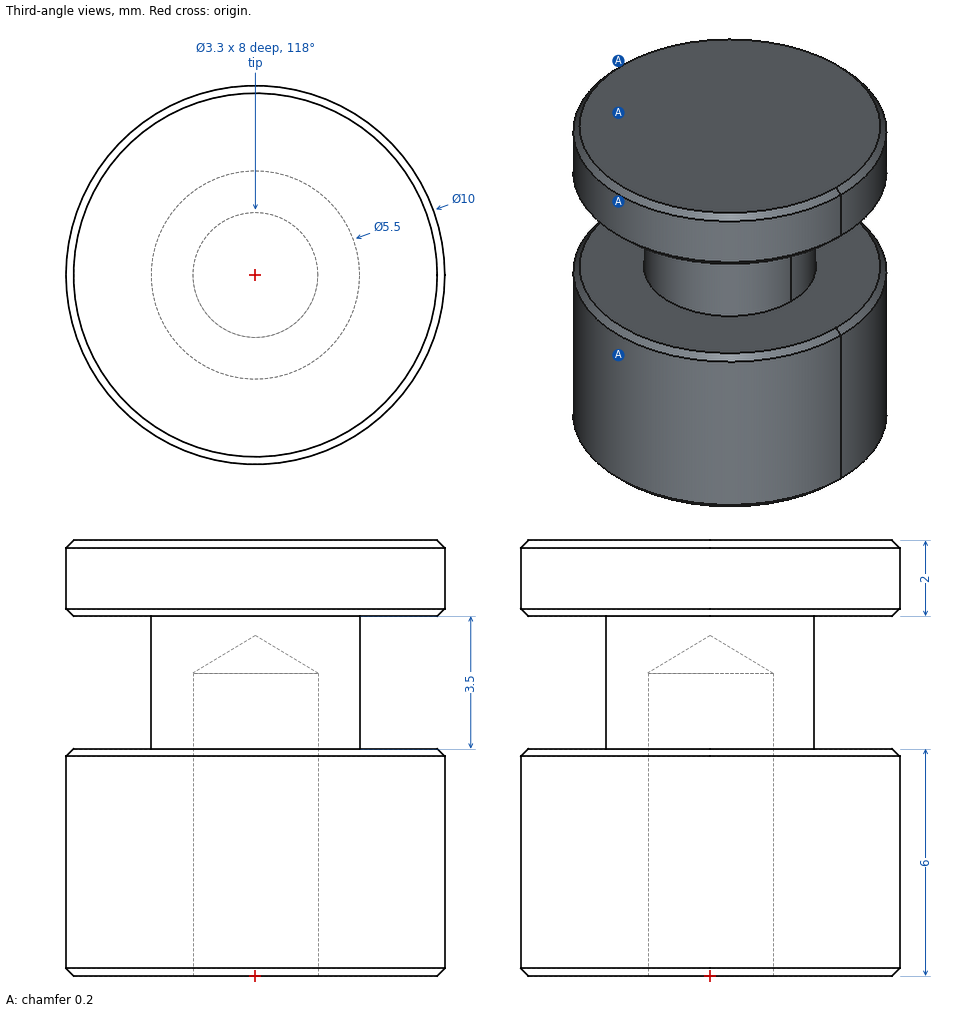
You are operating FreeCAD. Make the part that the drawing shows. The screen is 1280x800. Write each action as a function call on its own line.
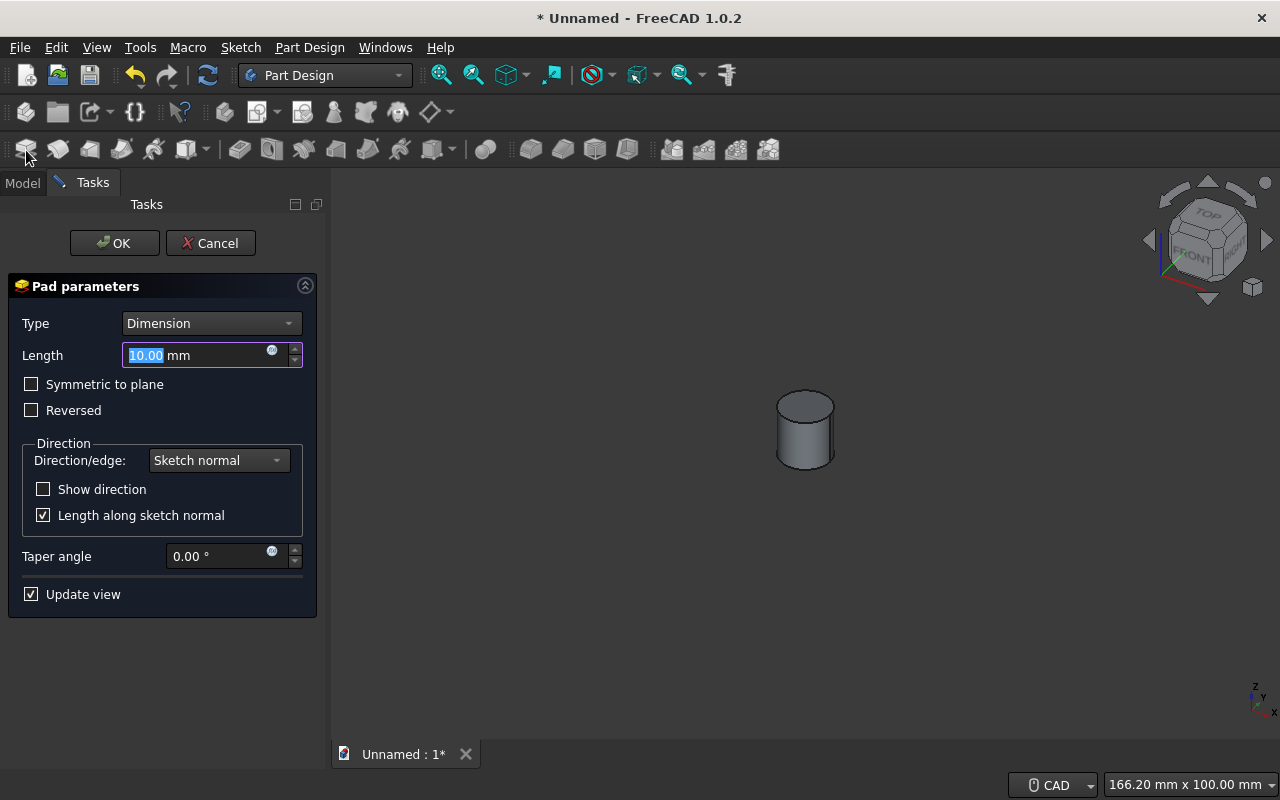
text(6)
key(Tab)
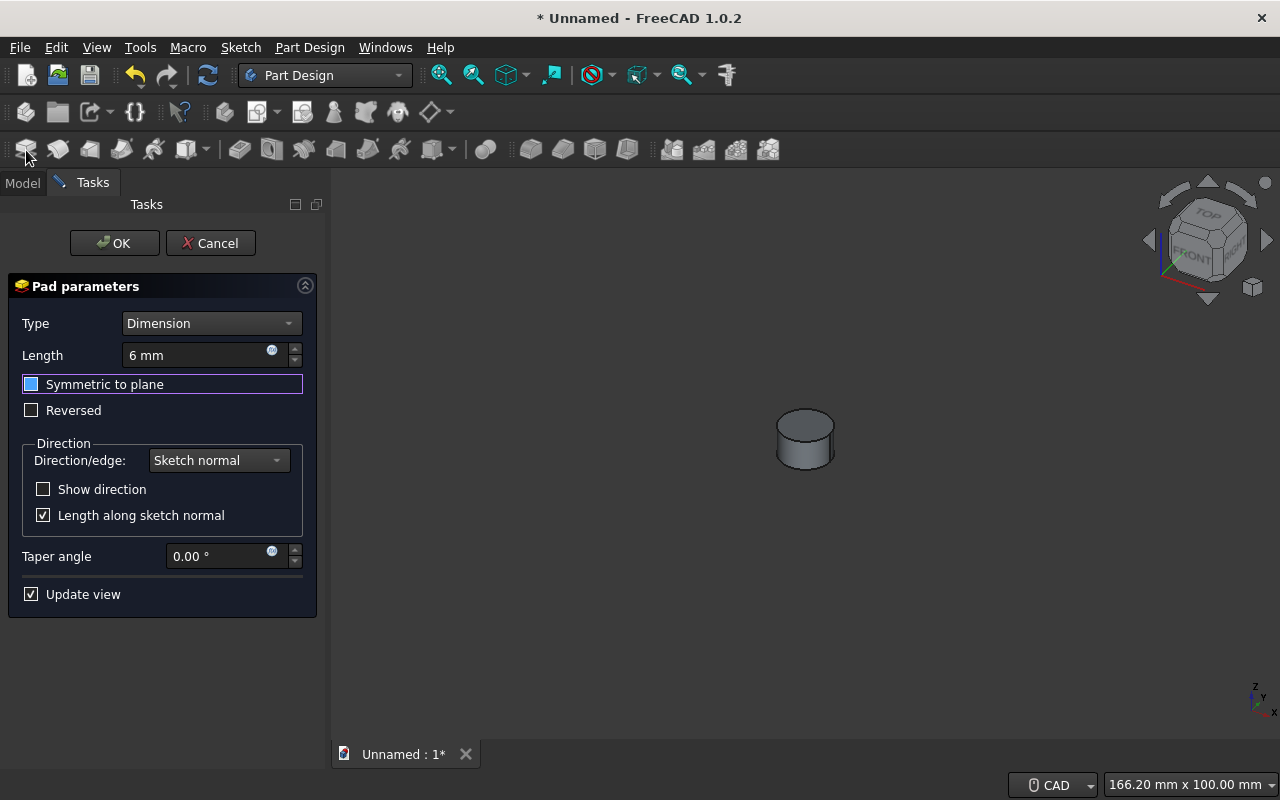
click(115, 243)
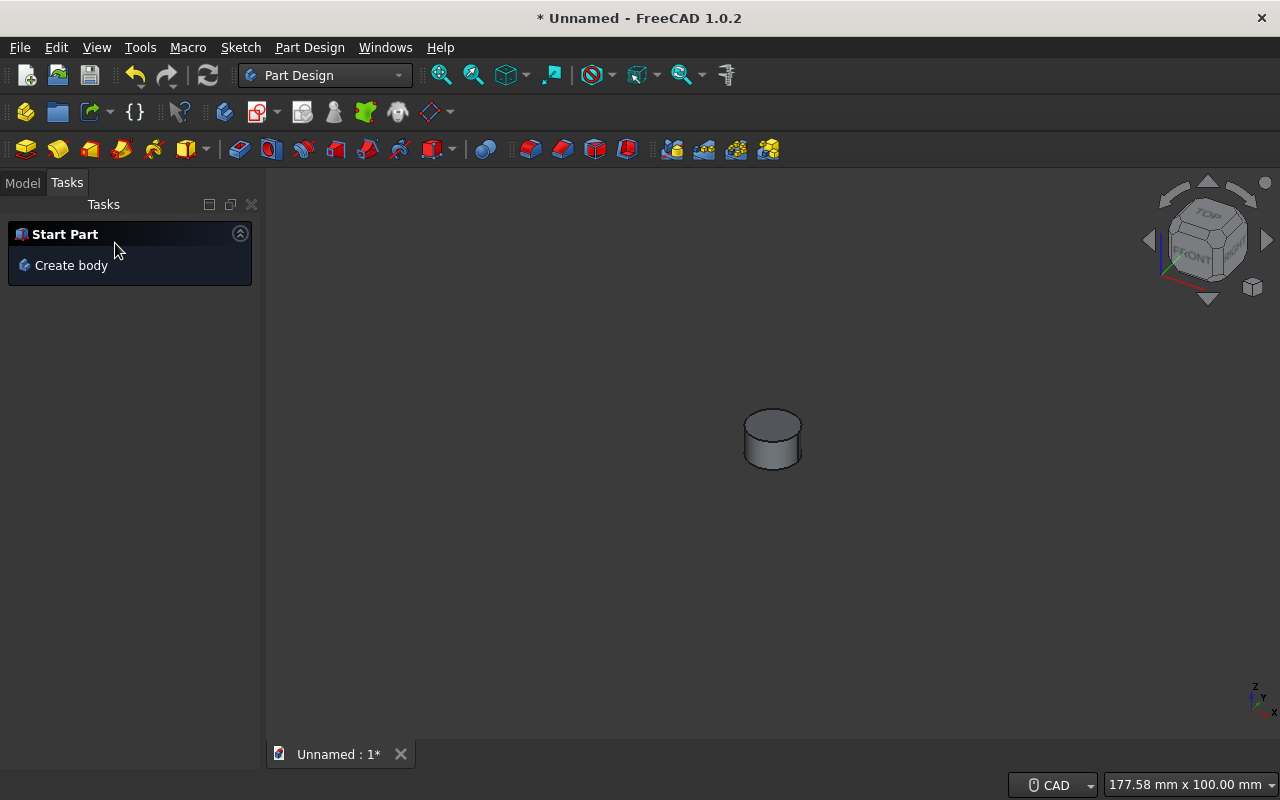
click(442, 76)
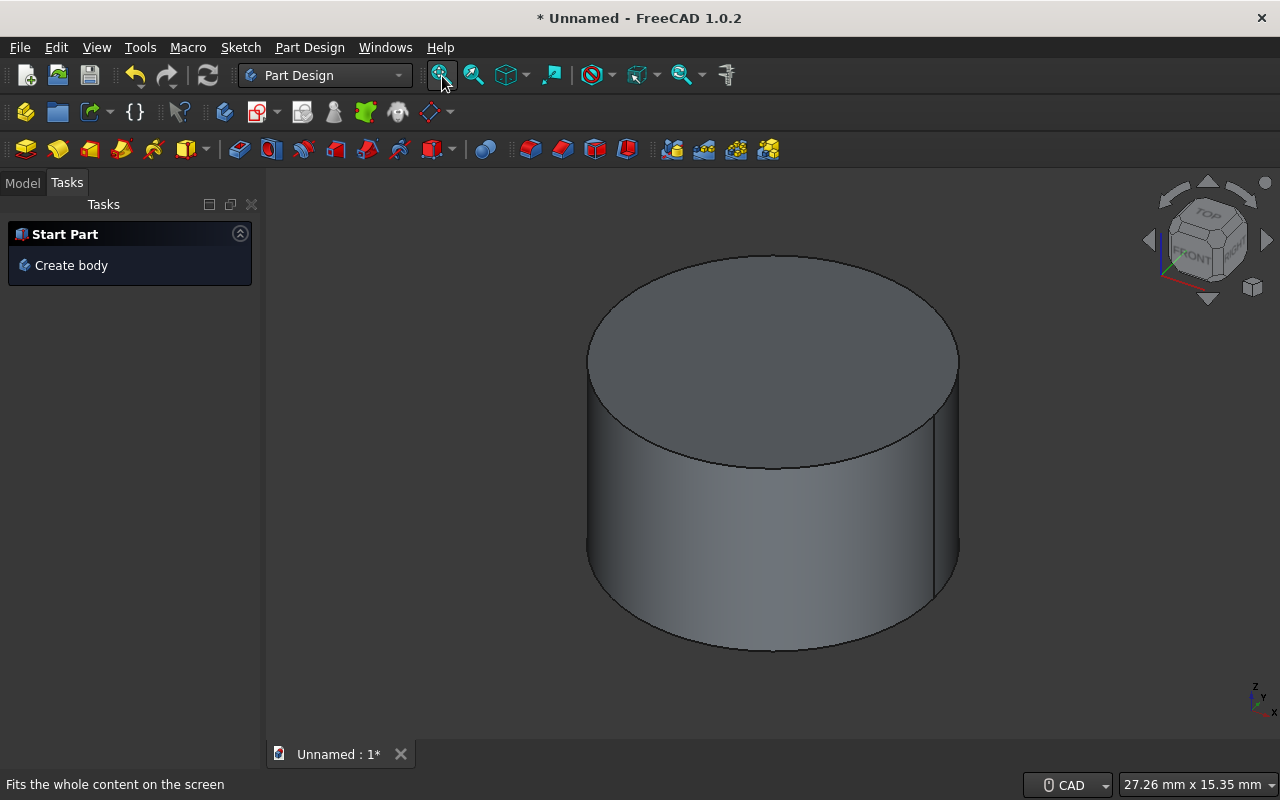
click(773, 361)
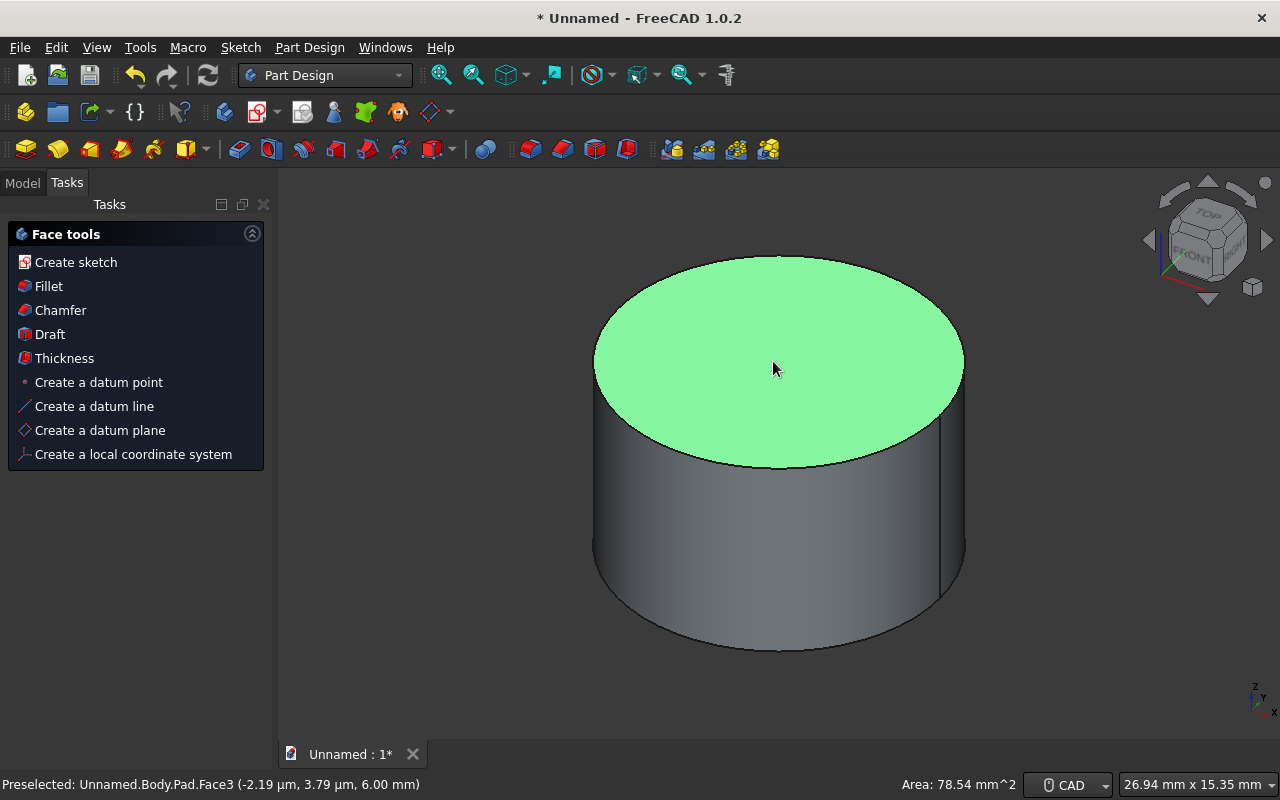
click(258, 112)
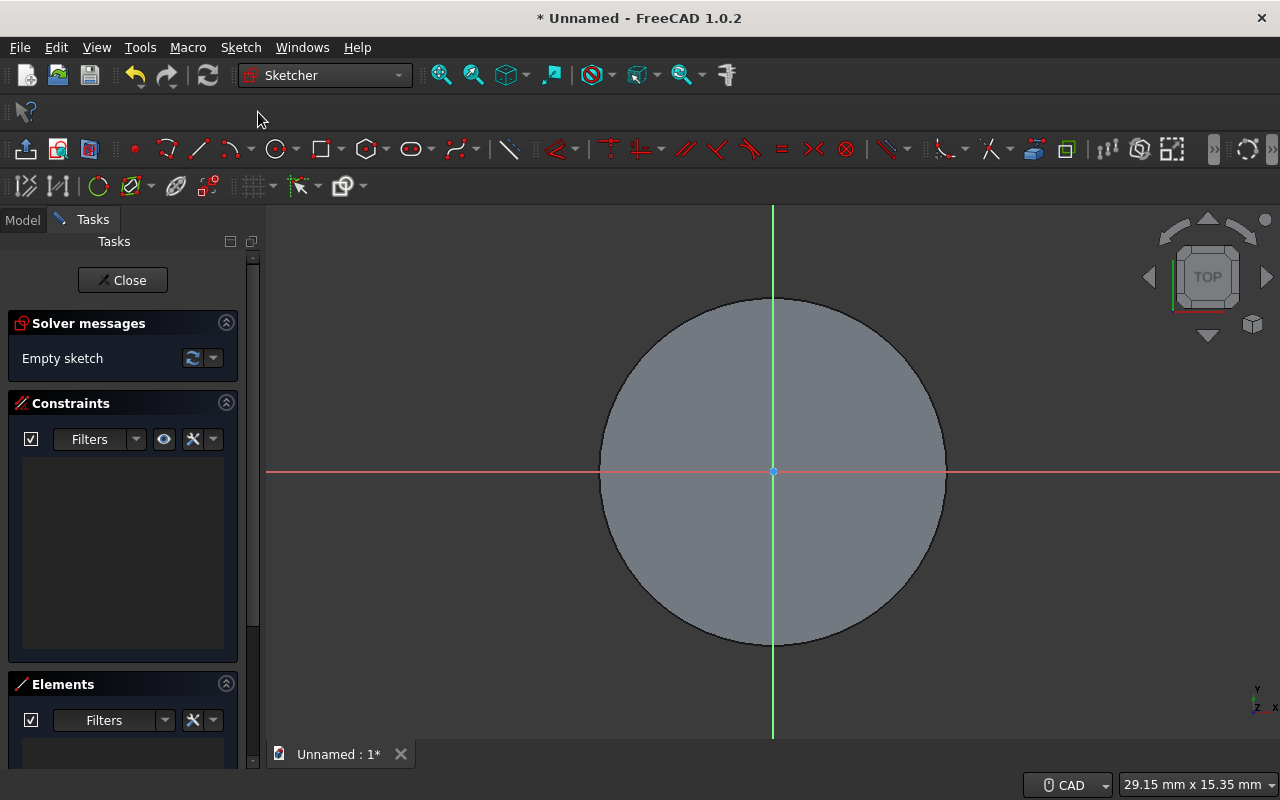
scroll(856, 472, up, 3)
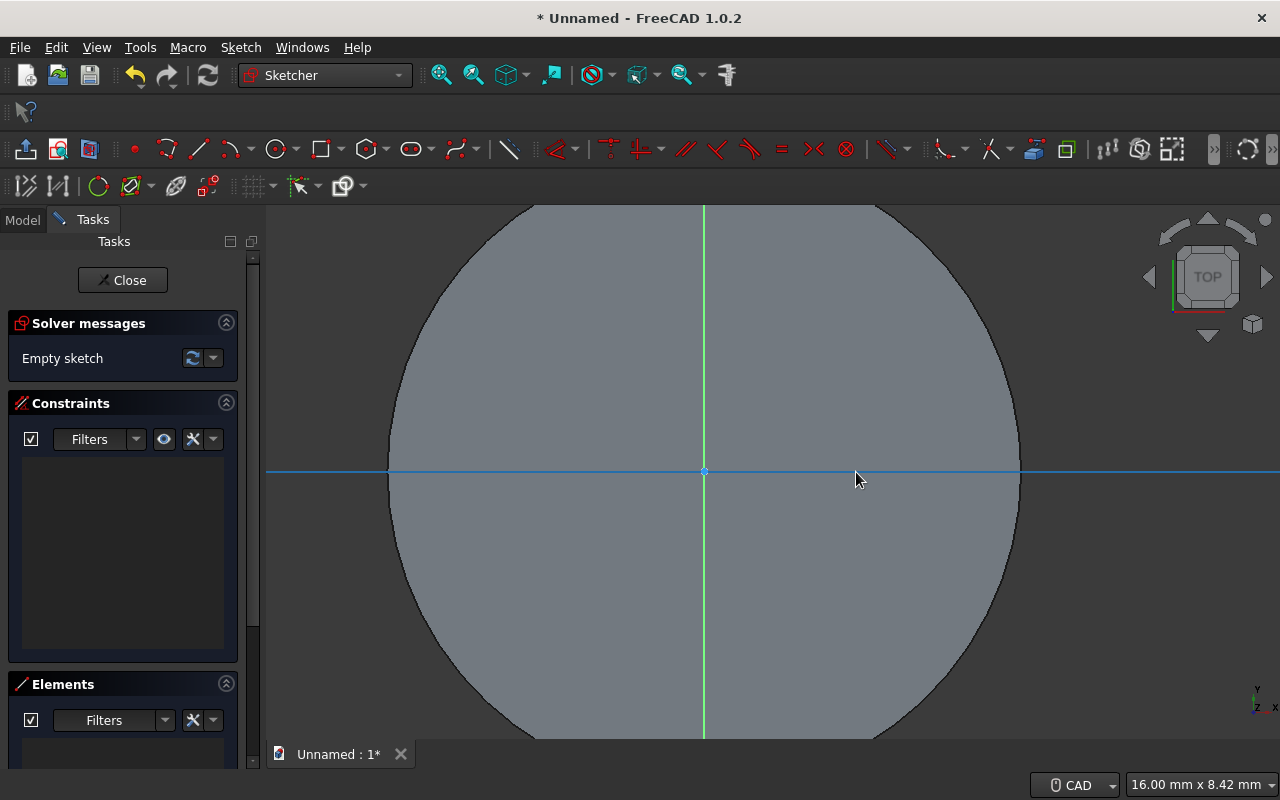
click(276, 150)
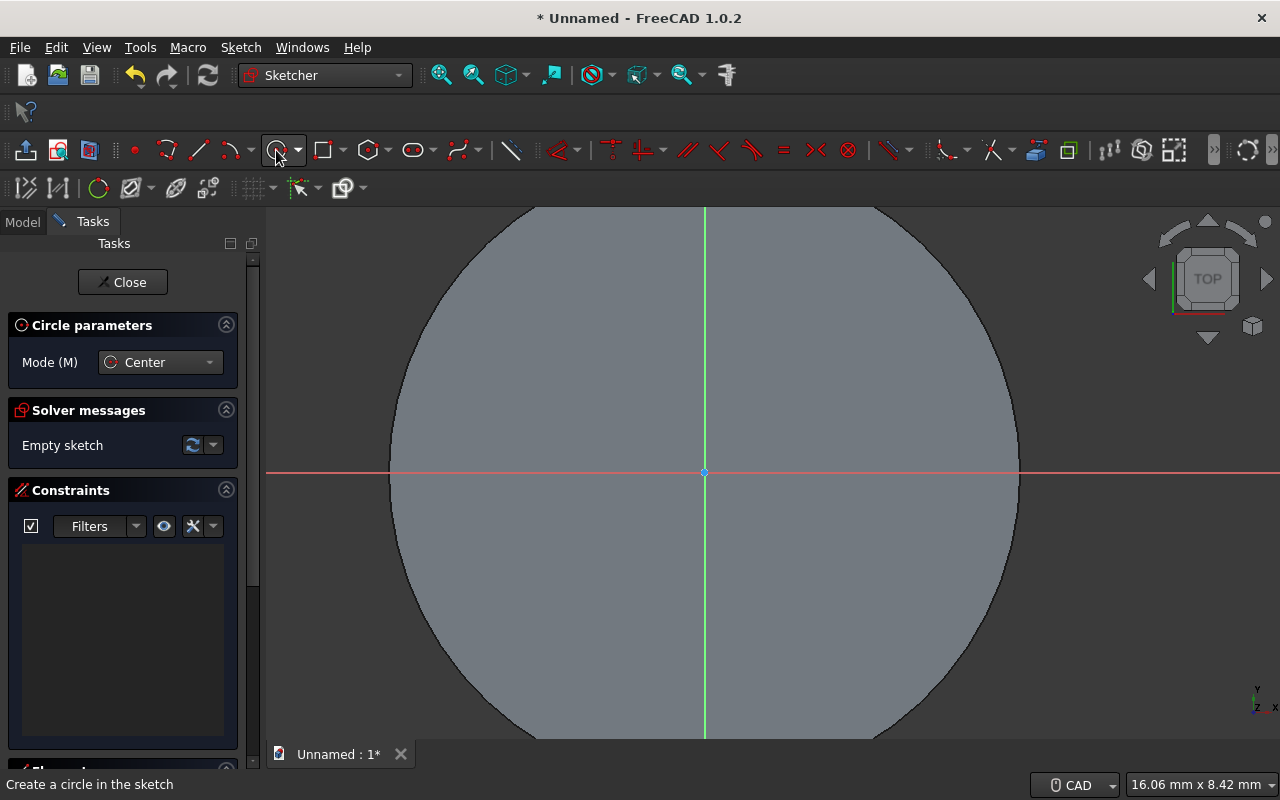
click(705, 473)
move(827, 350)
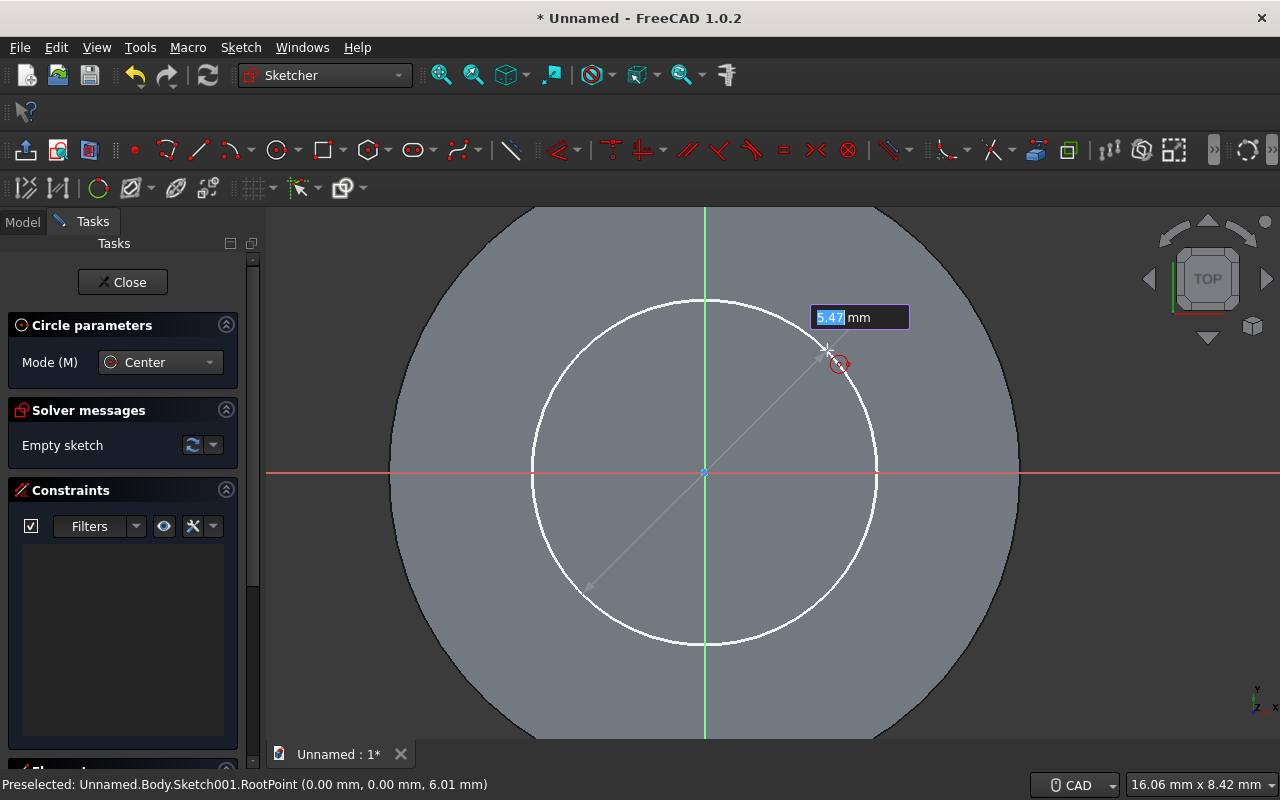
text(5.5)
key(Return)
key(Escape)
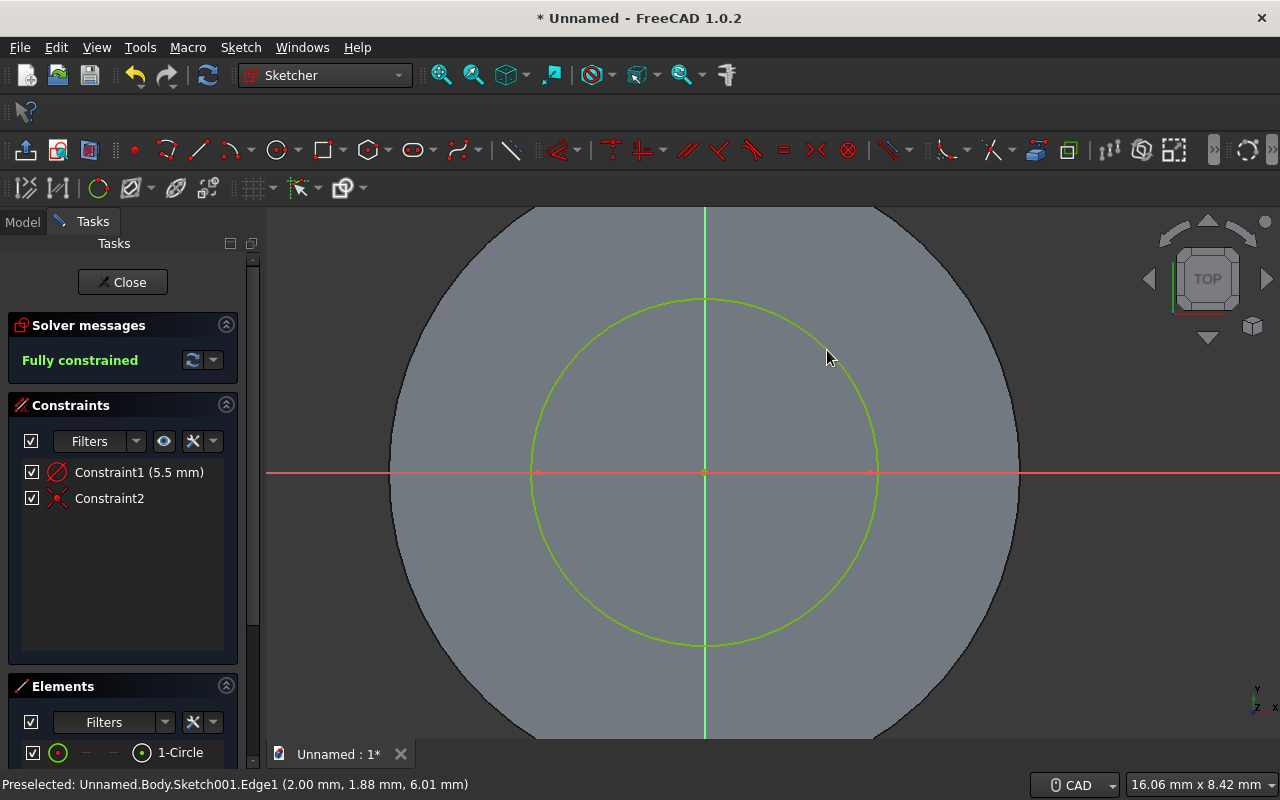
click(123, 282)